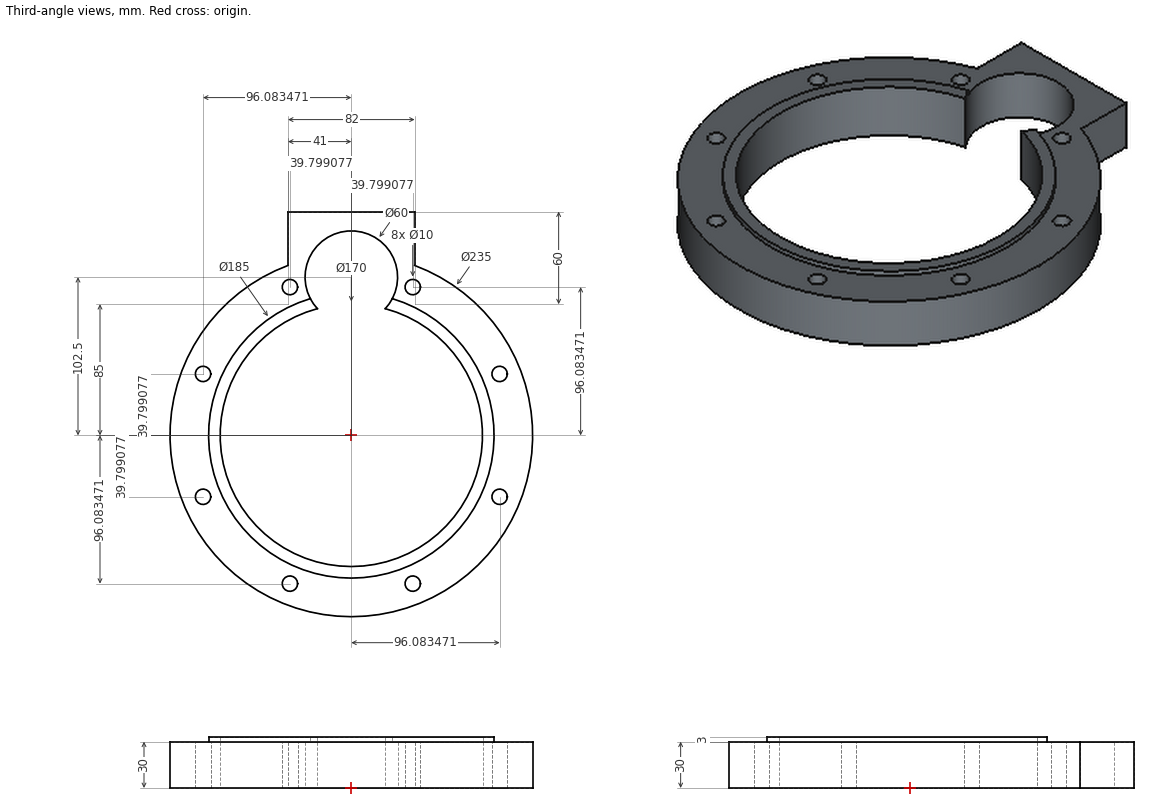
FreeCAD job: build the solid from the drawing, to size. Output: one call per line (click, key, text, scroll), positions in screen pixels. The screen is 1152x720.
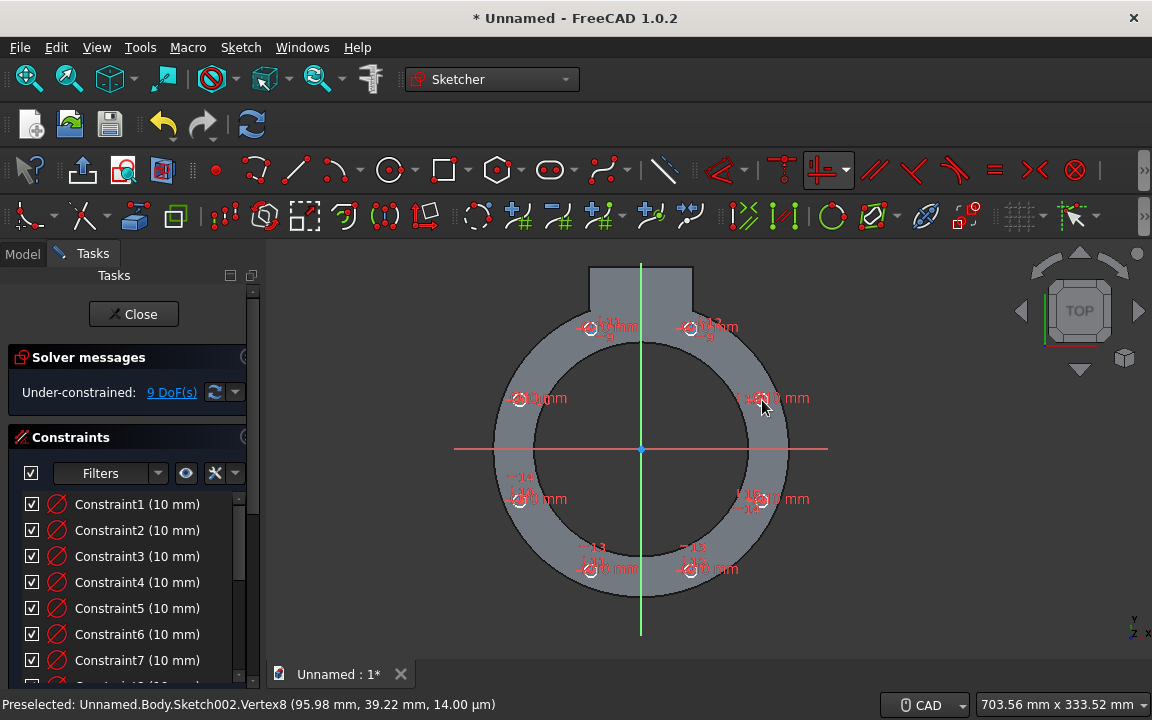
click(848, 170)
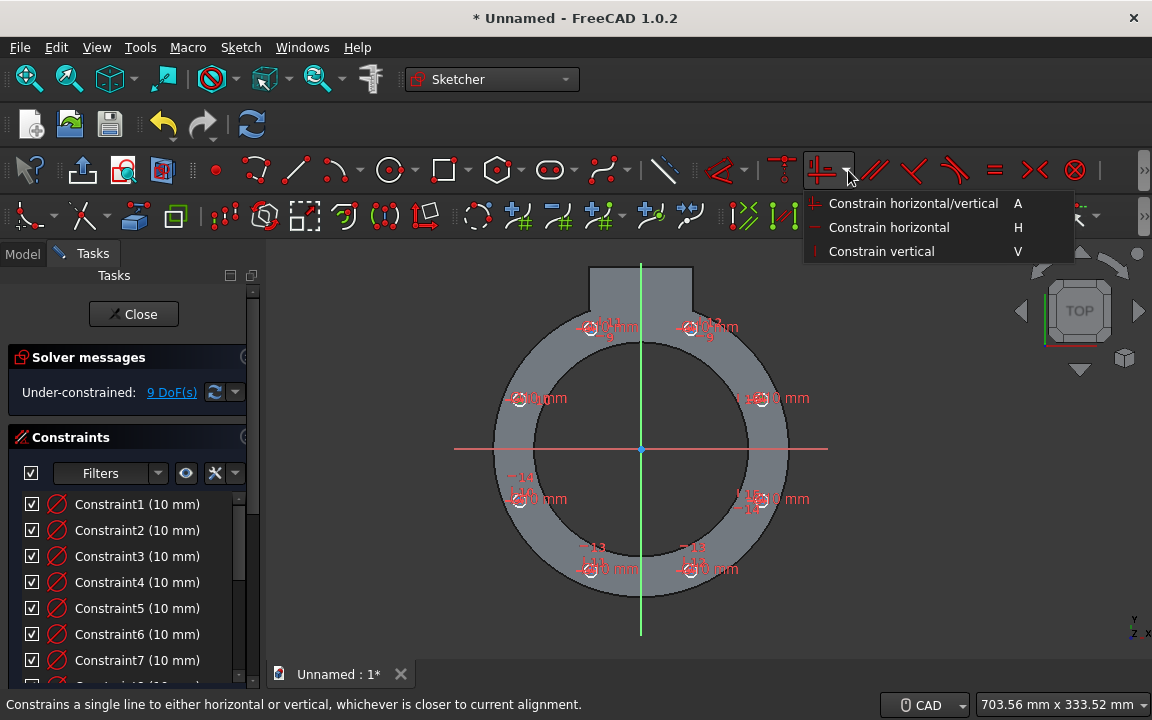
click(939, 227)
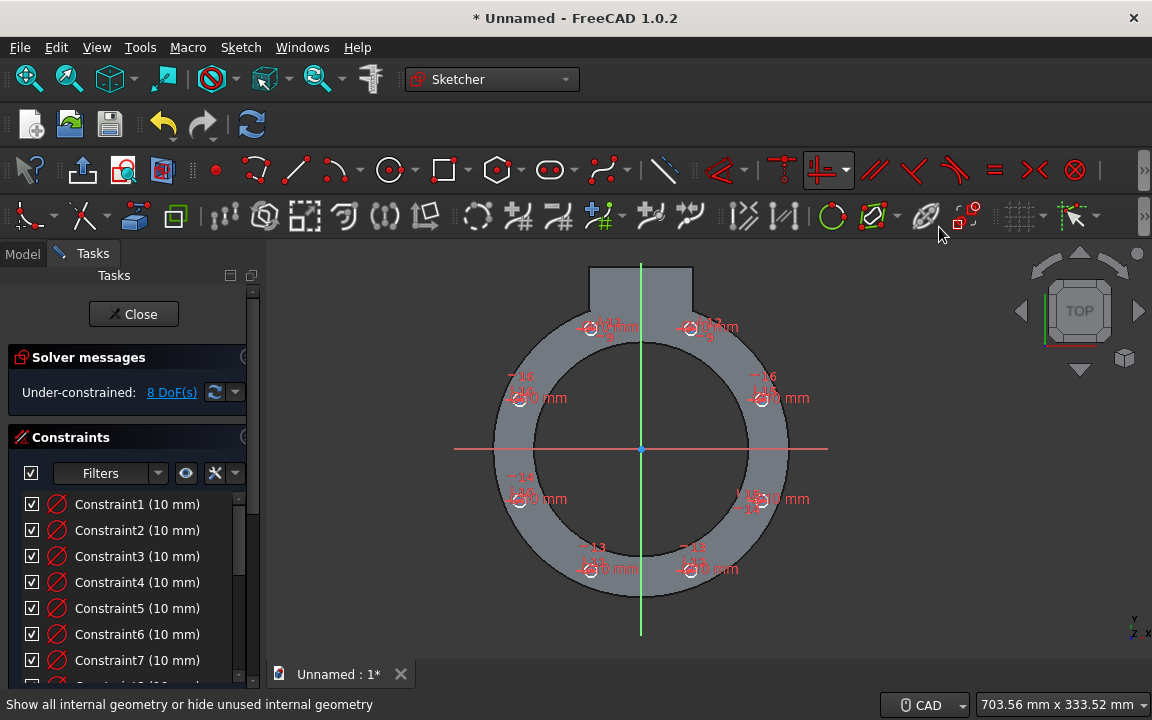
click(691, 329)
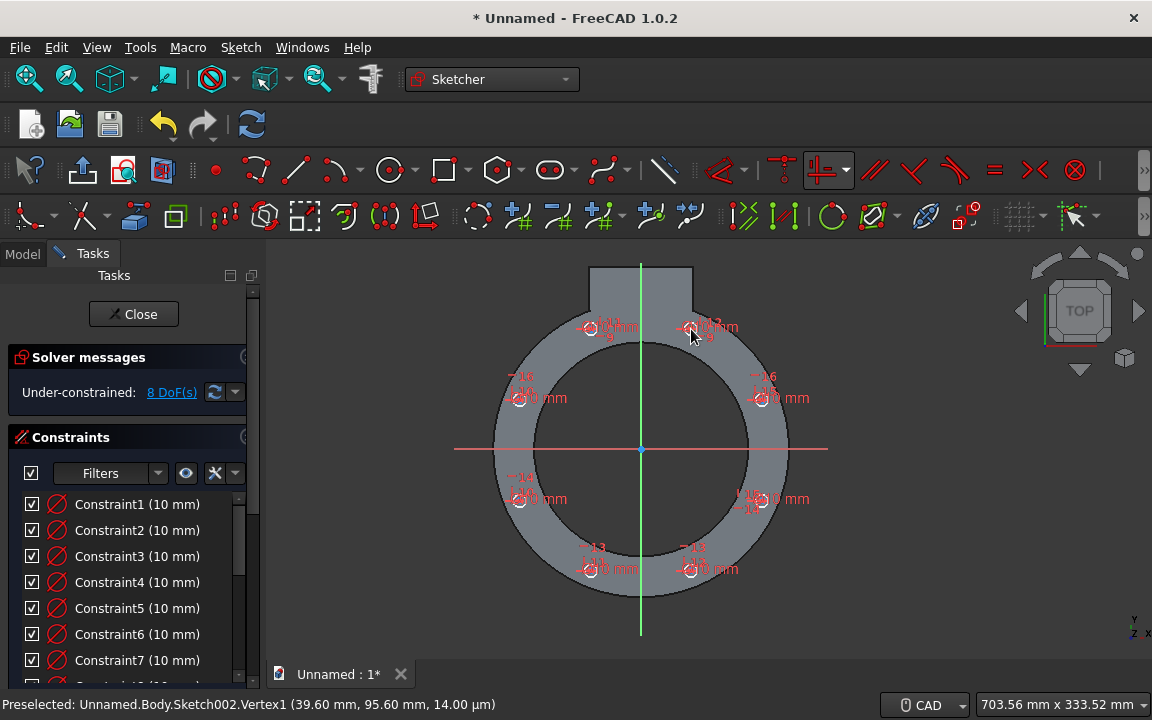
click(746, 170)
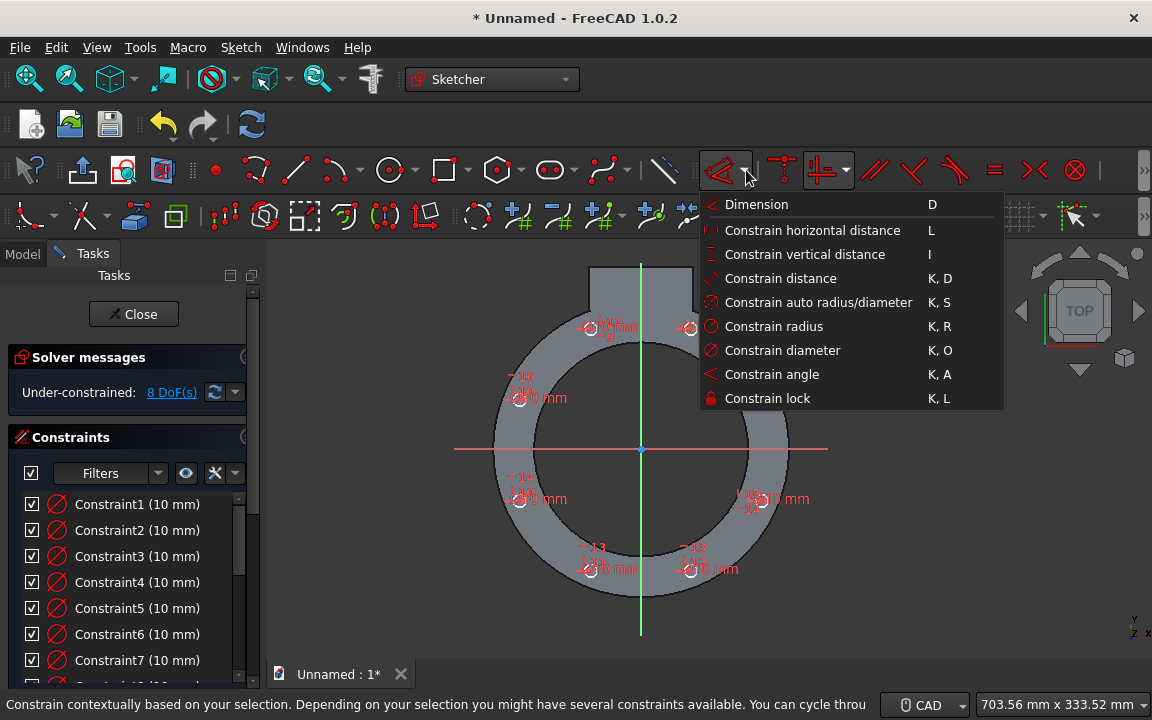
click(852, 230)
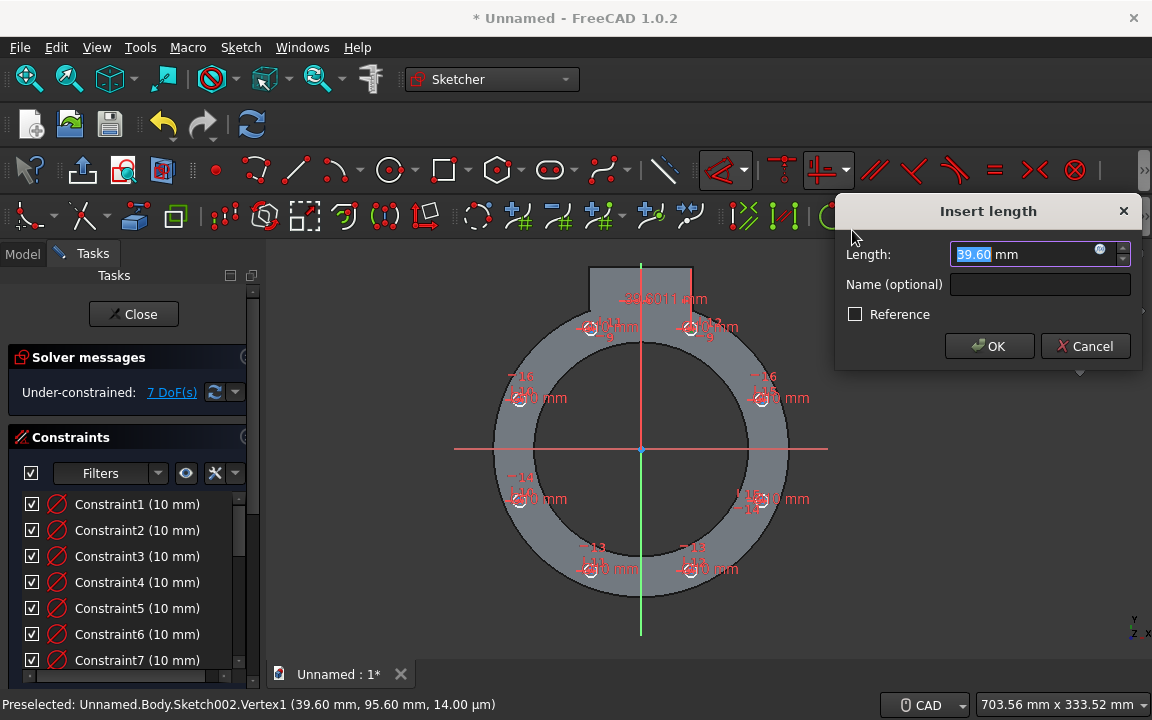
text(39.799077)
key(Return)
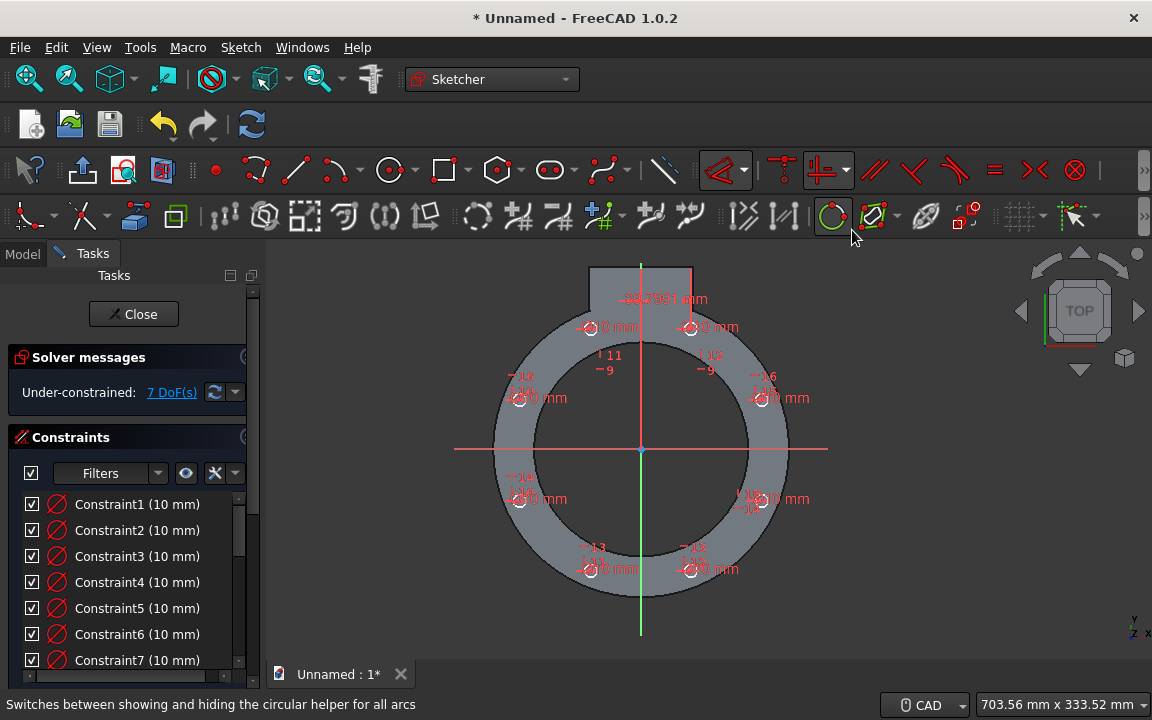
click(691, 329)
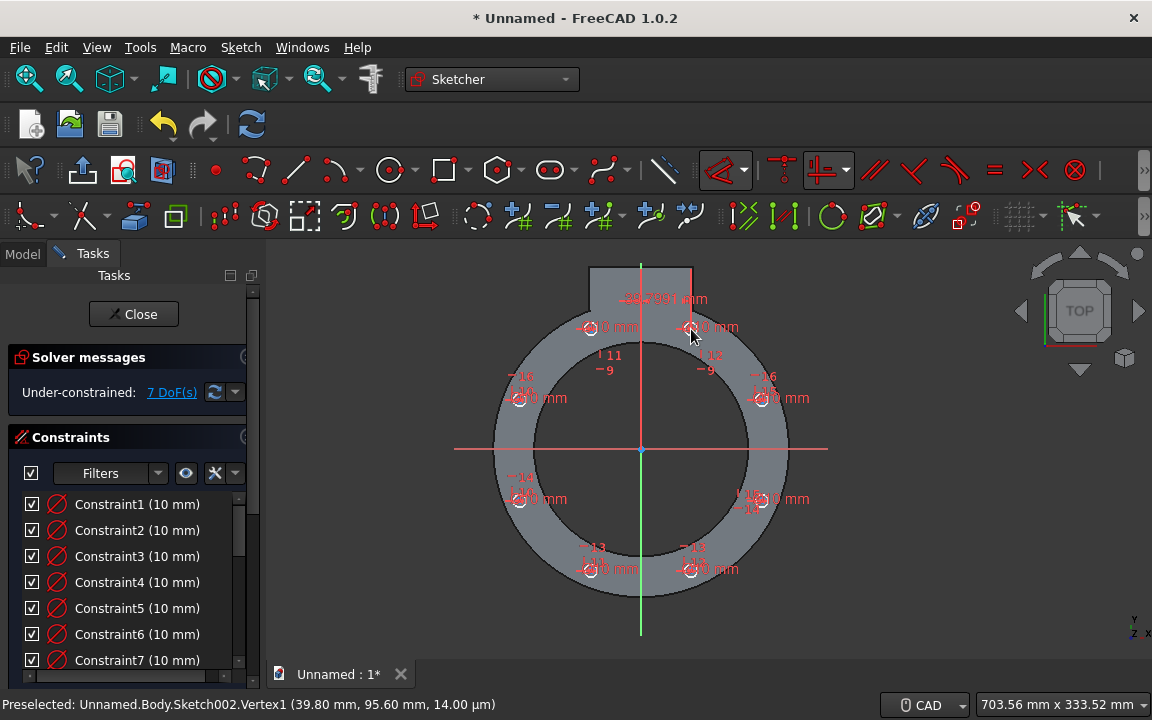
key(i)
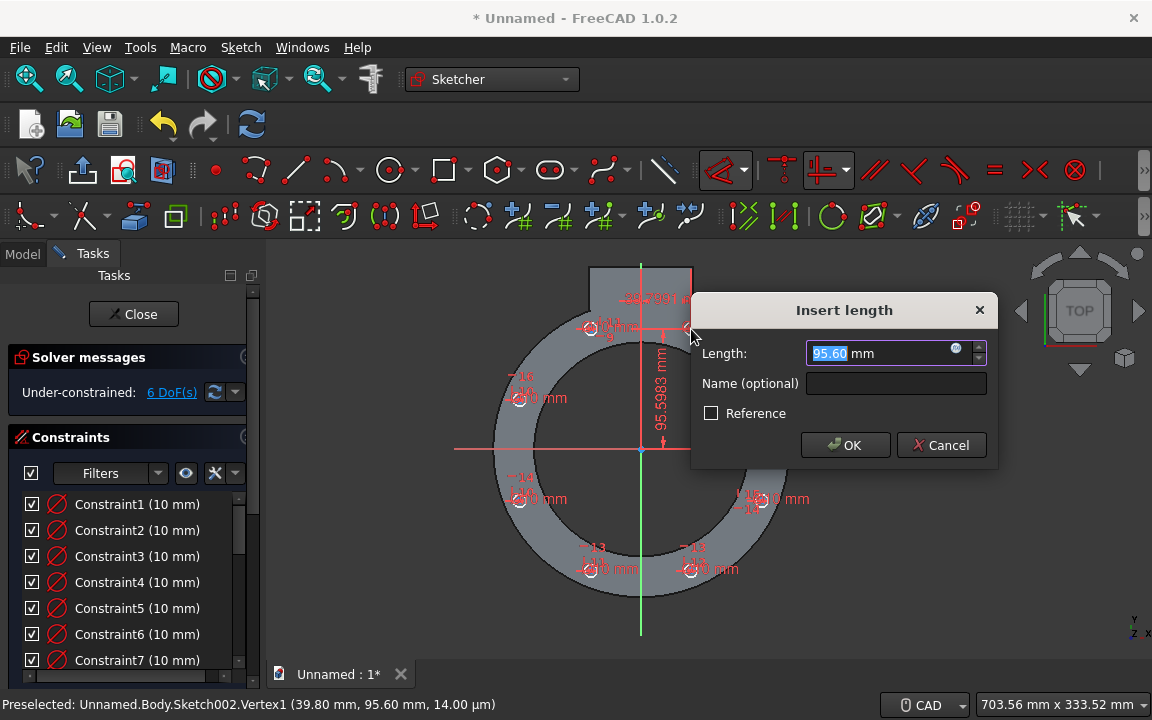
text(96.083471)
key(Return)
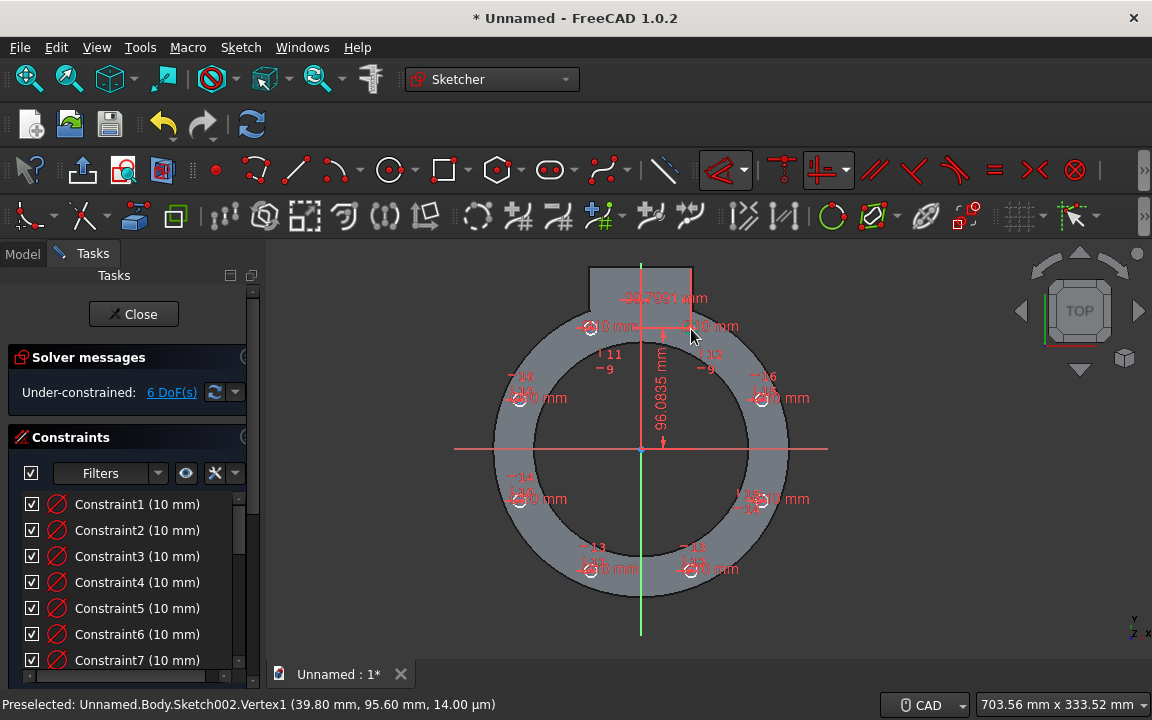
click(591, 328)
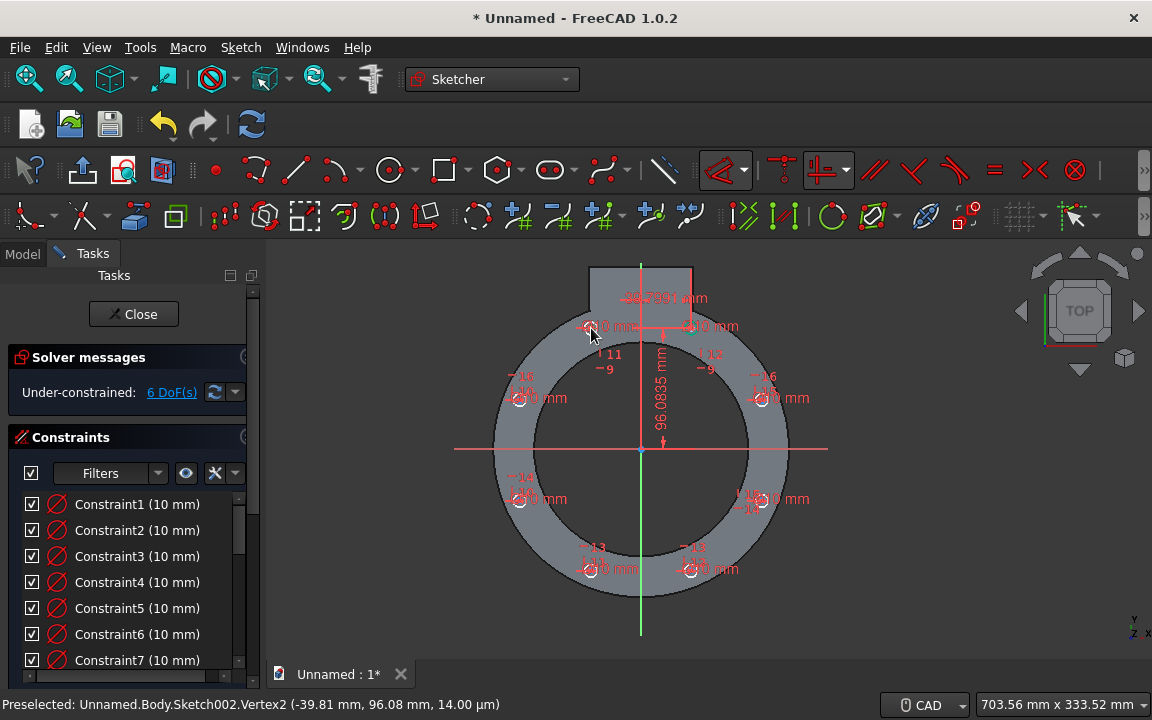
key(l)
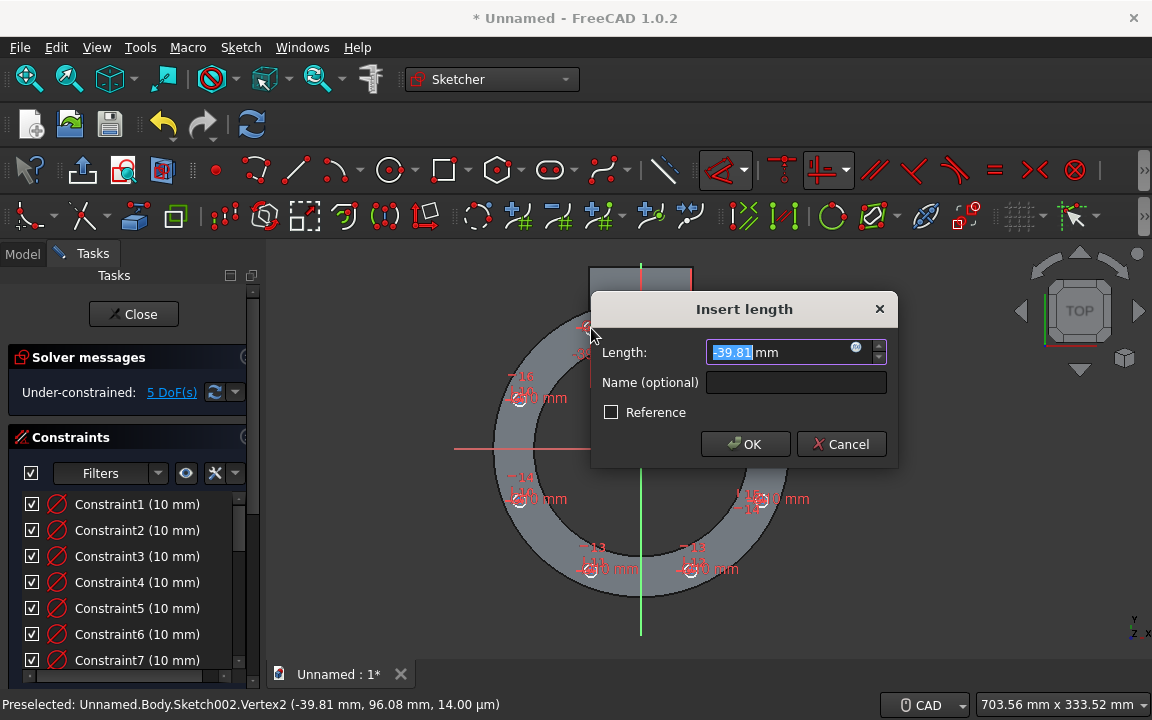
text(-39.799077)
key(Return)